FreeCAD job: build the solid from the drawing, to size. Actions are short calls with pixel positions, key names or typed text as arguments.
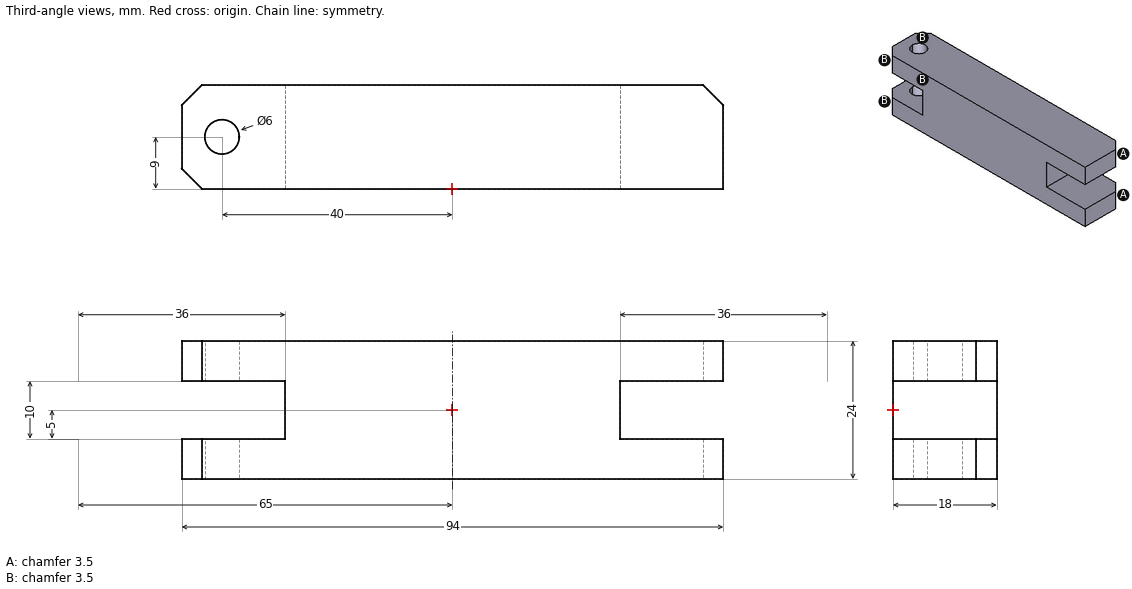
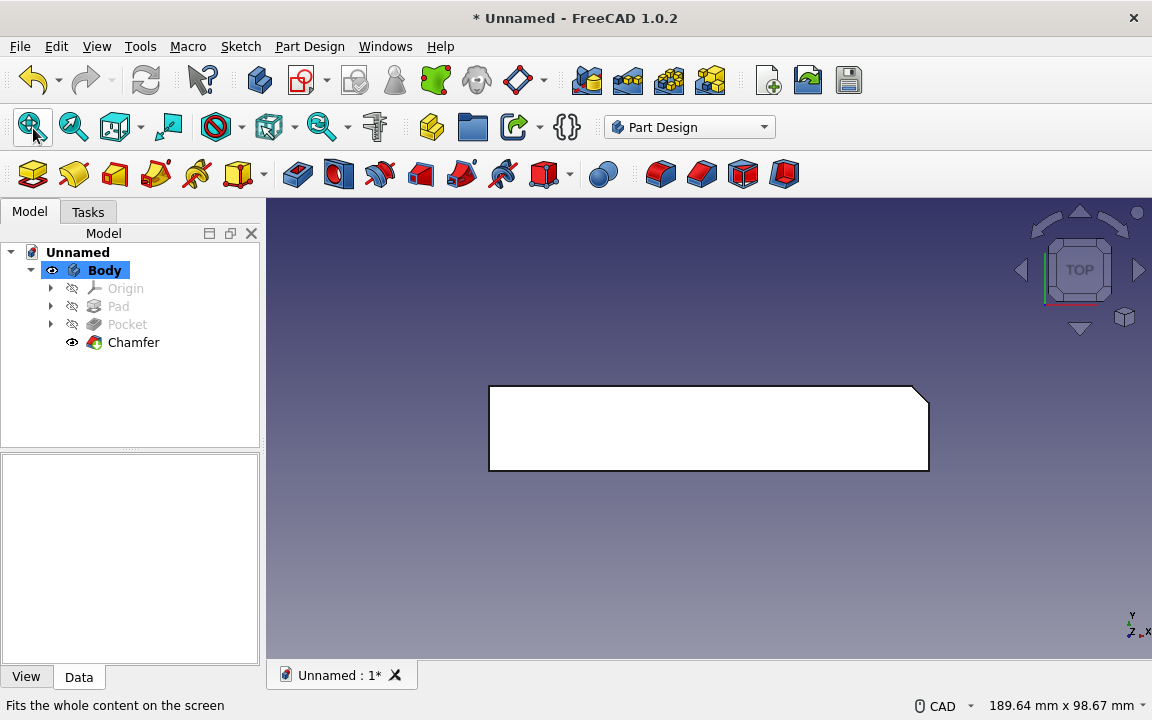
key(1)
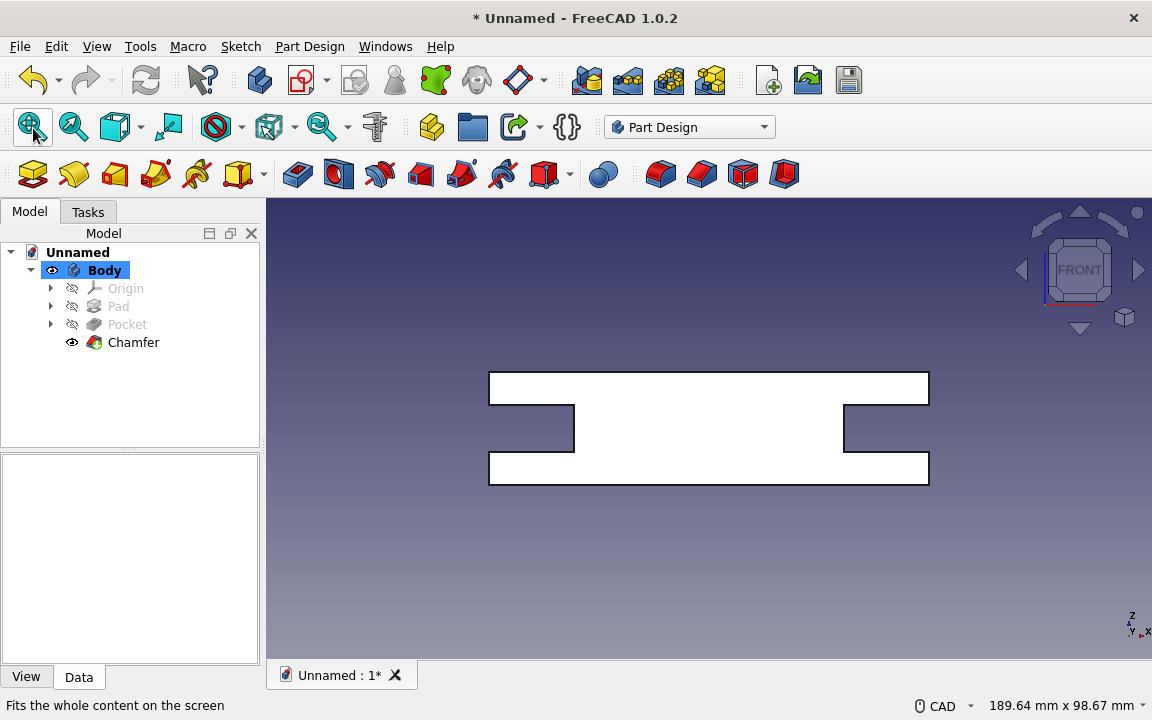
click(489, 467)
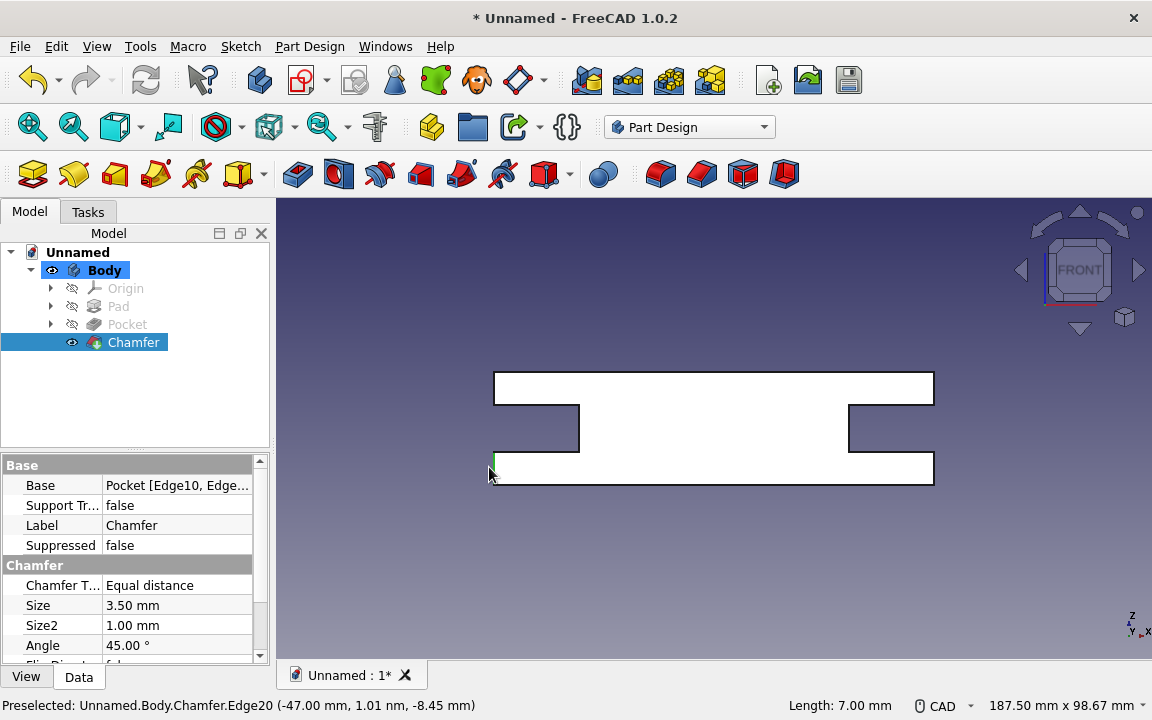
key(3)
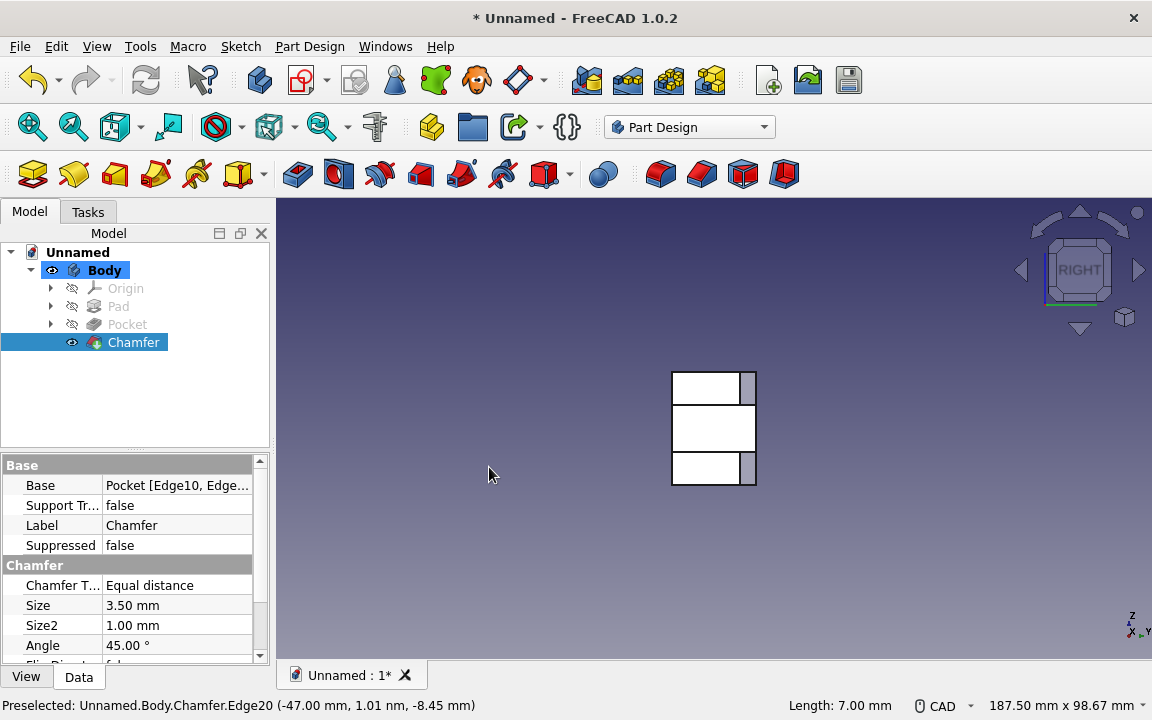
key(v)
key(f)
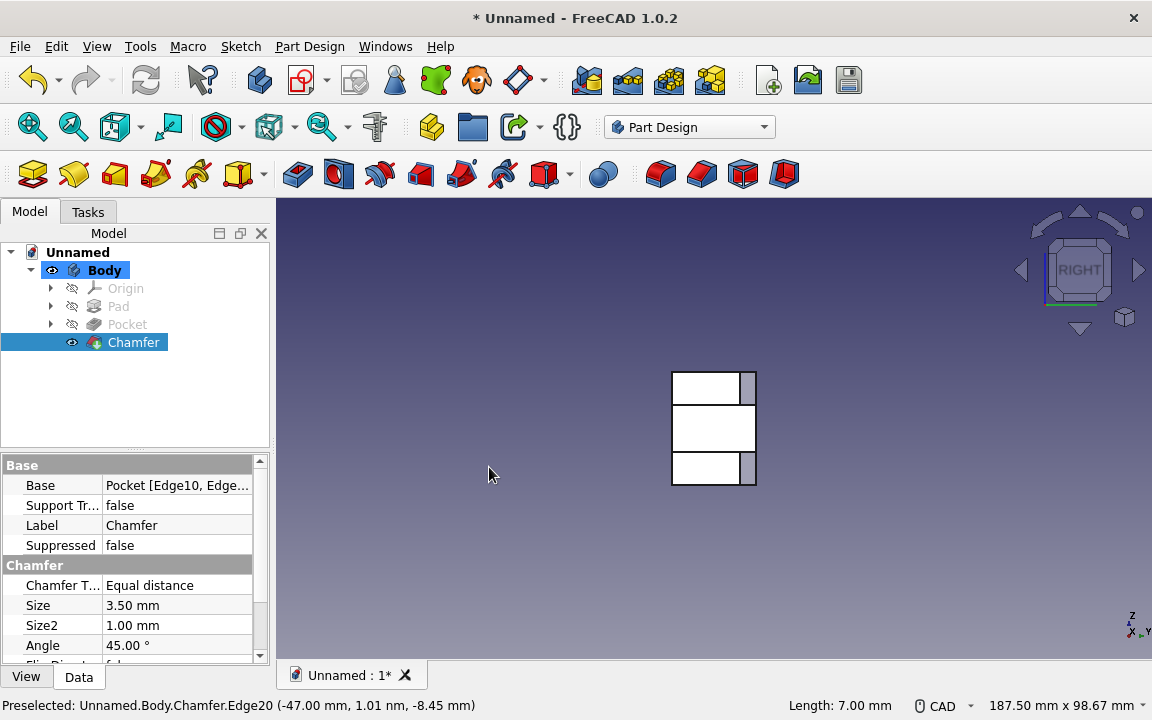
key(5)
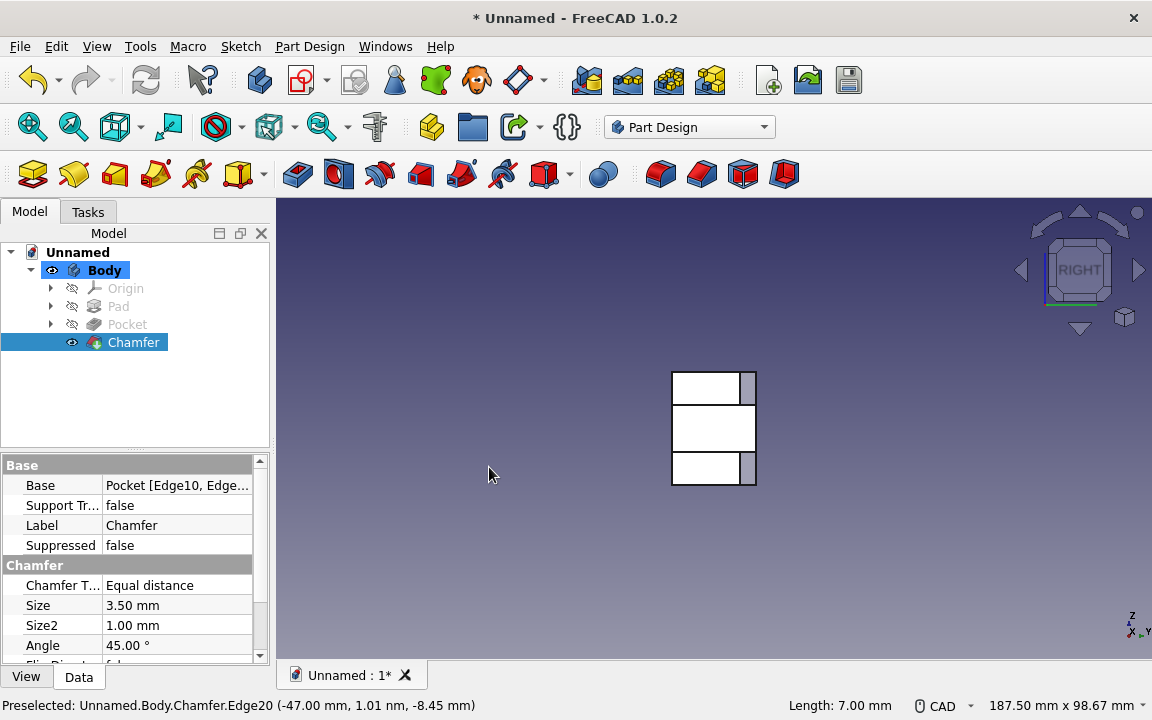
key(4)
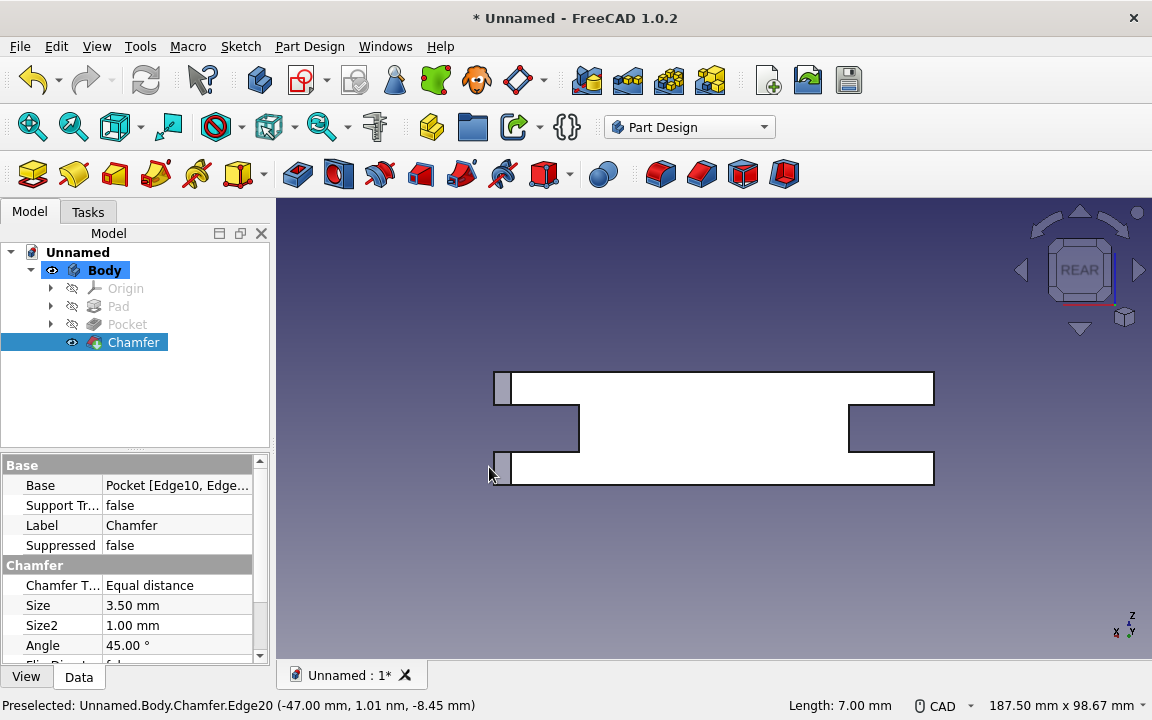
click(934, 467, ctrl)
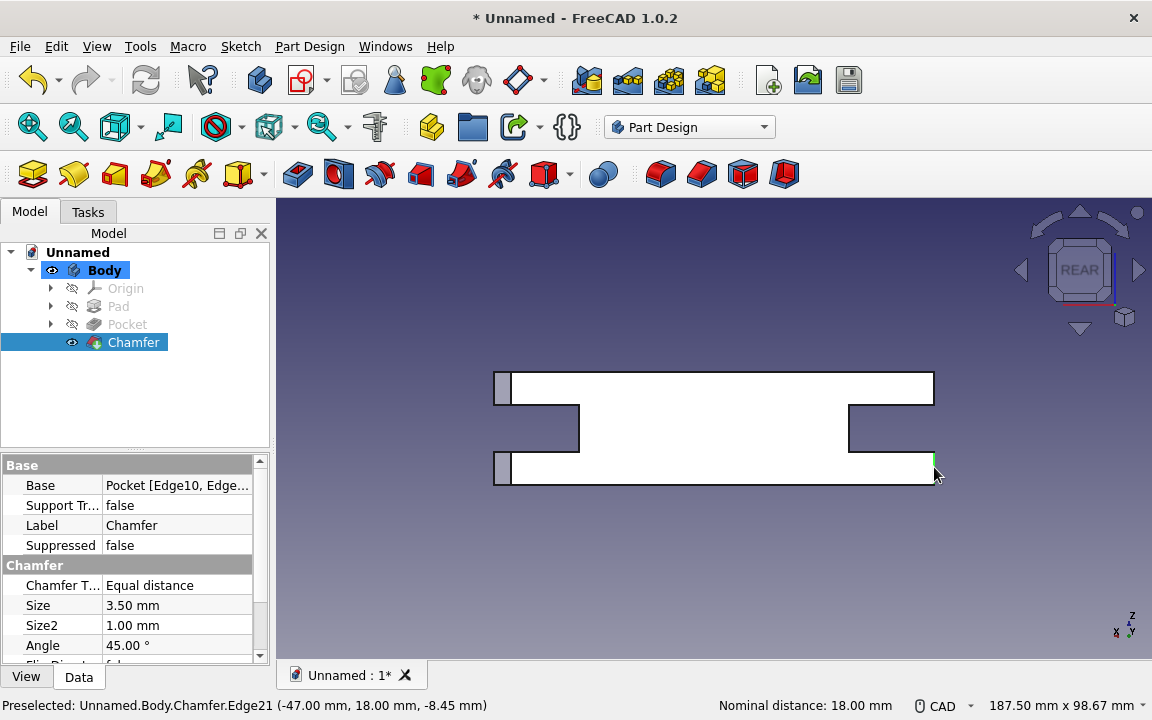
click(934, 388, ctrl)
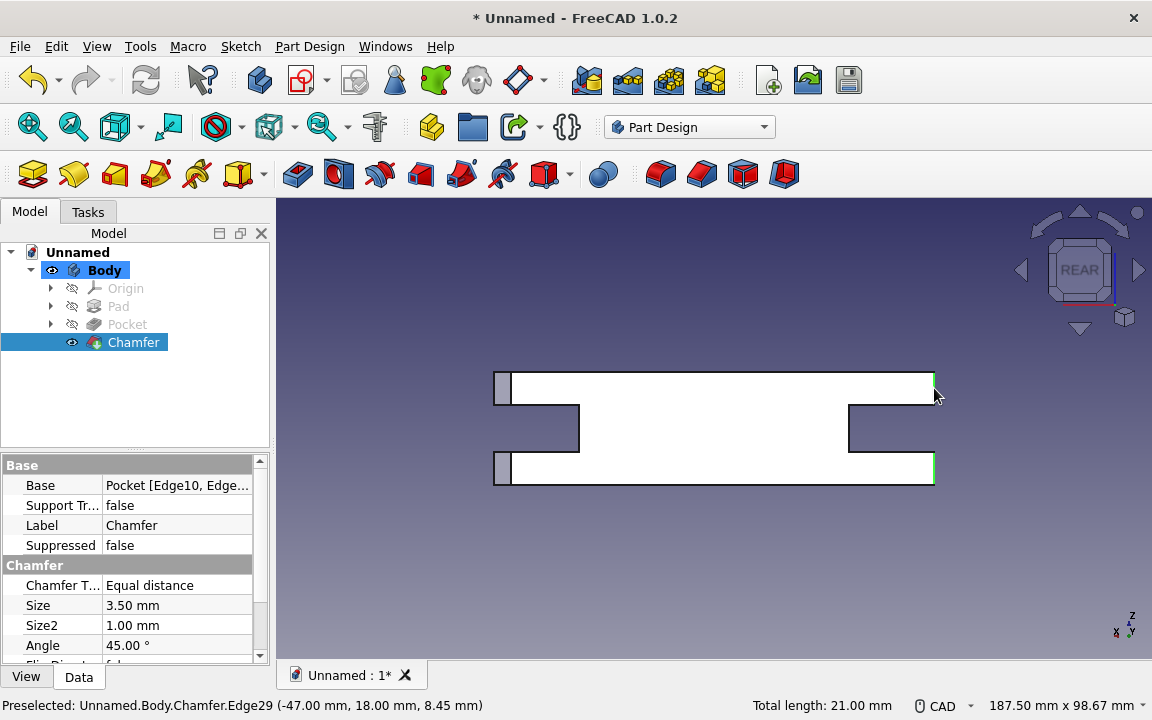
key(6)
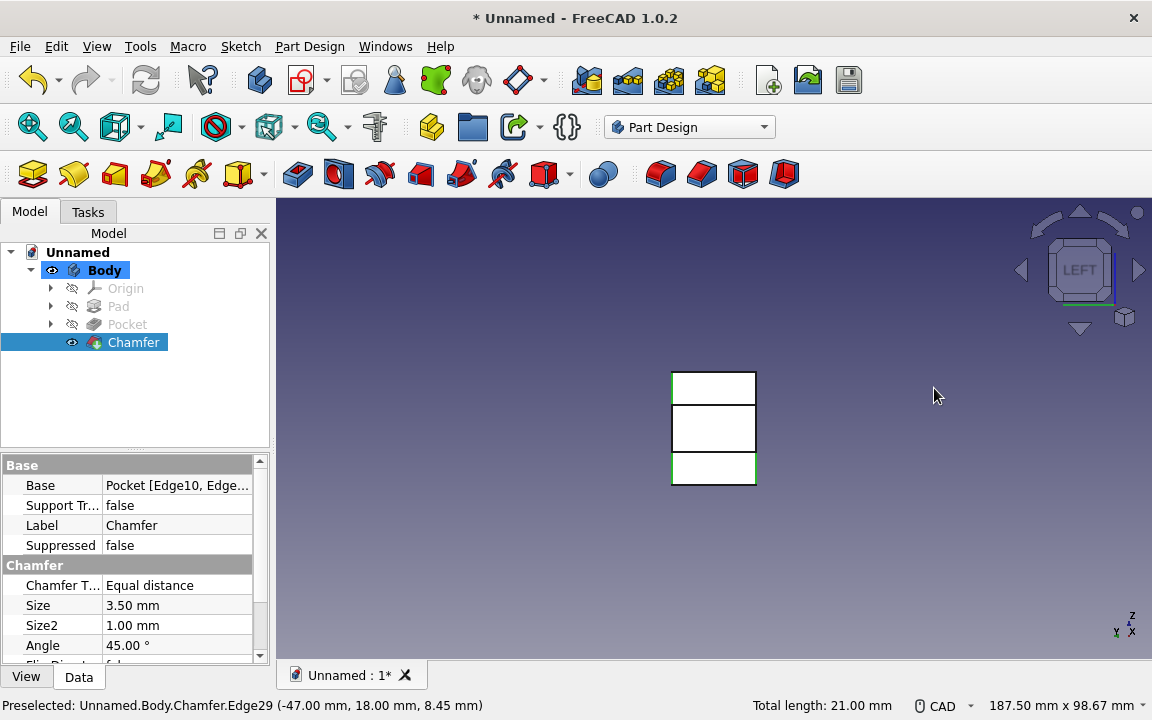
key(v)
key(f)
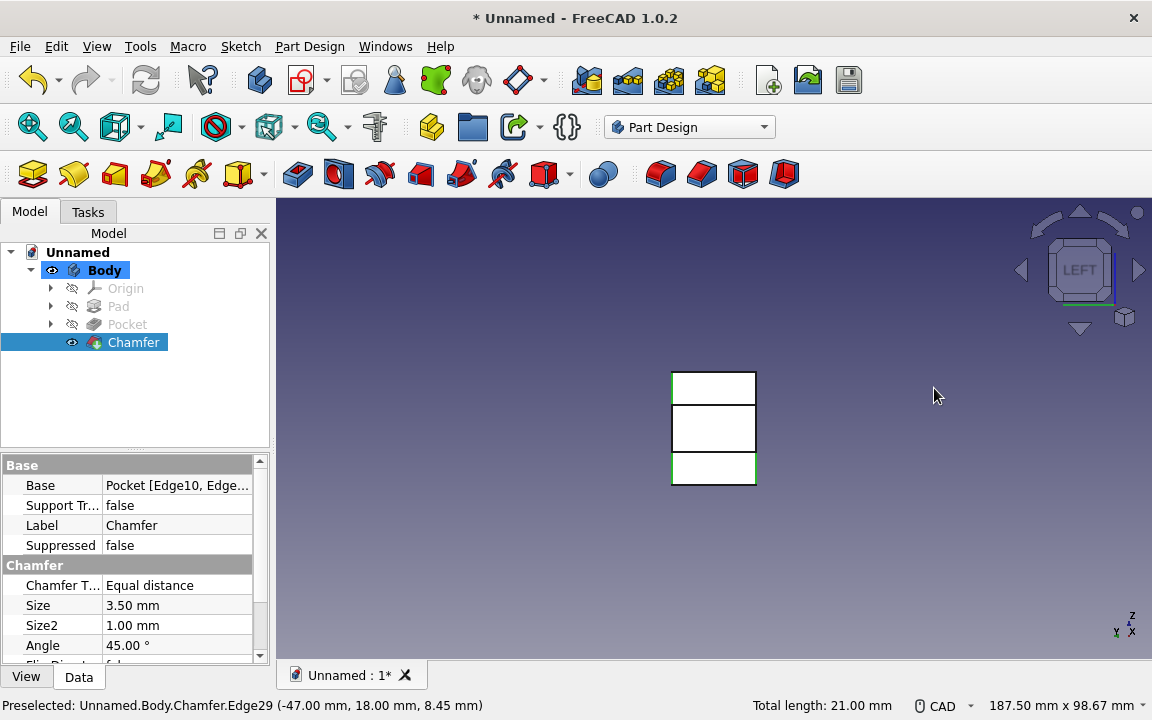
click(756, 388, ctrl)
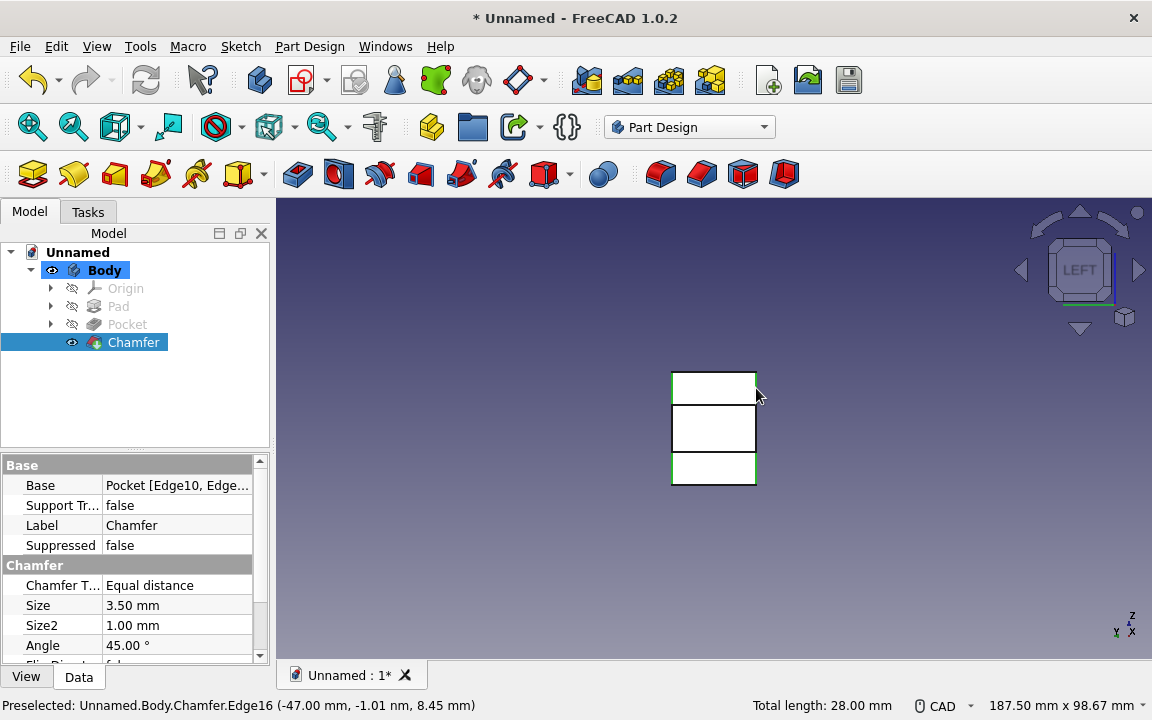
click(702, 174)